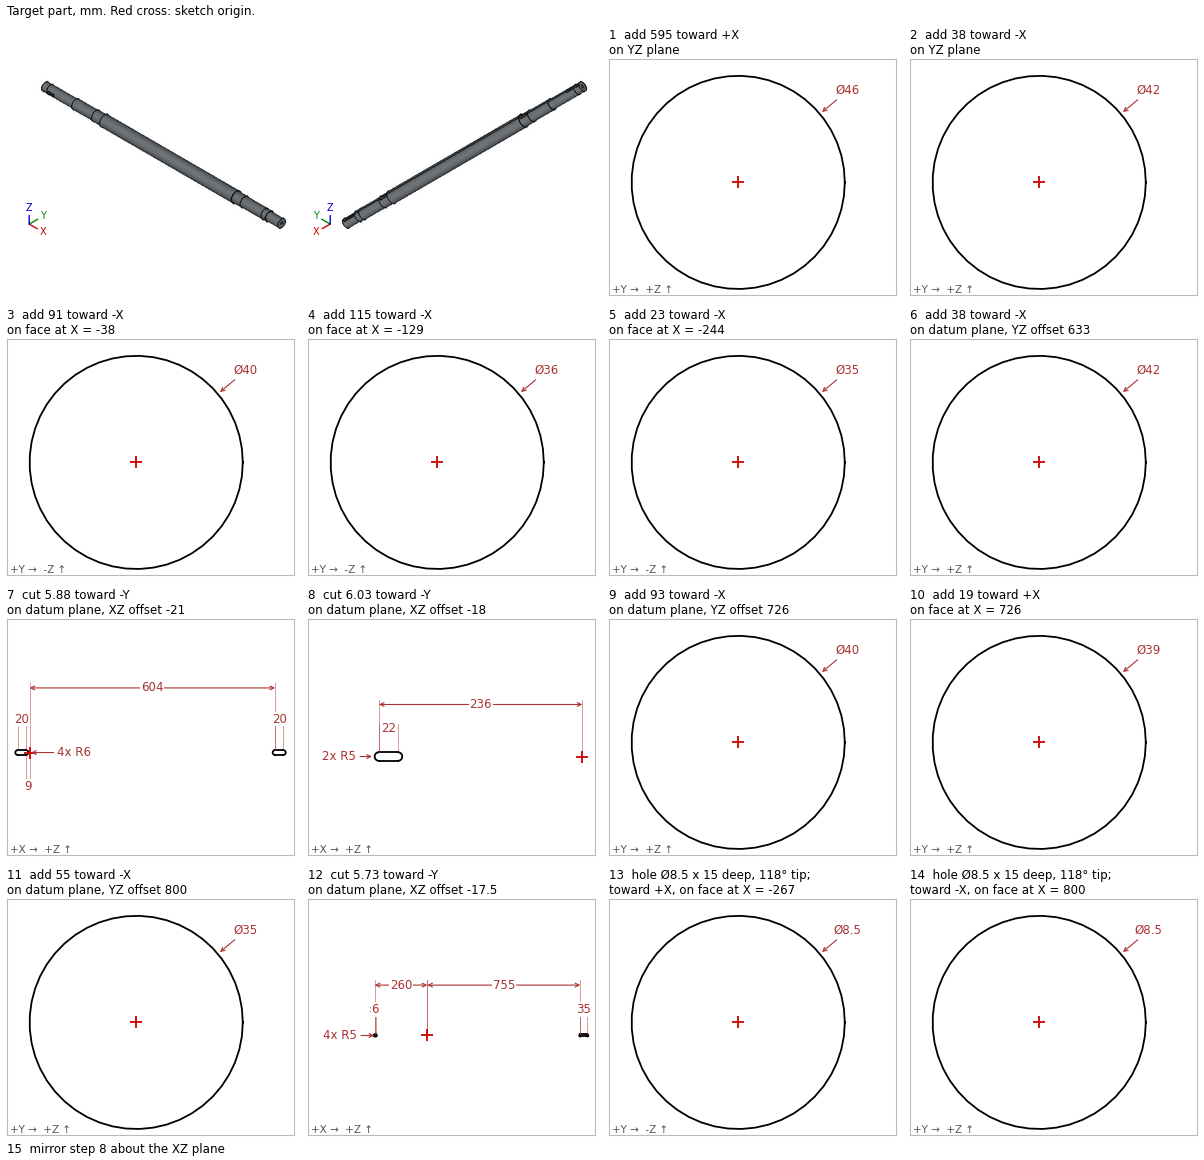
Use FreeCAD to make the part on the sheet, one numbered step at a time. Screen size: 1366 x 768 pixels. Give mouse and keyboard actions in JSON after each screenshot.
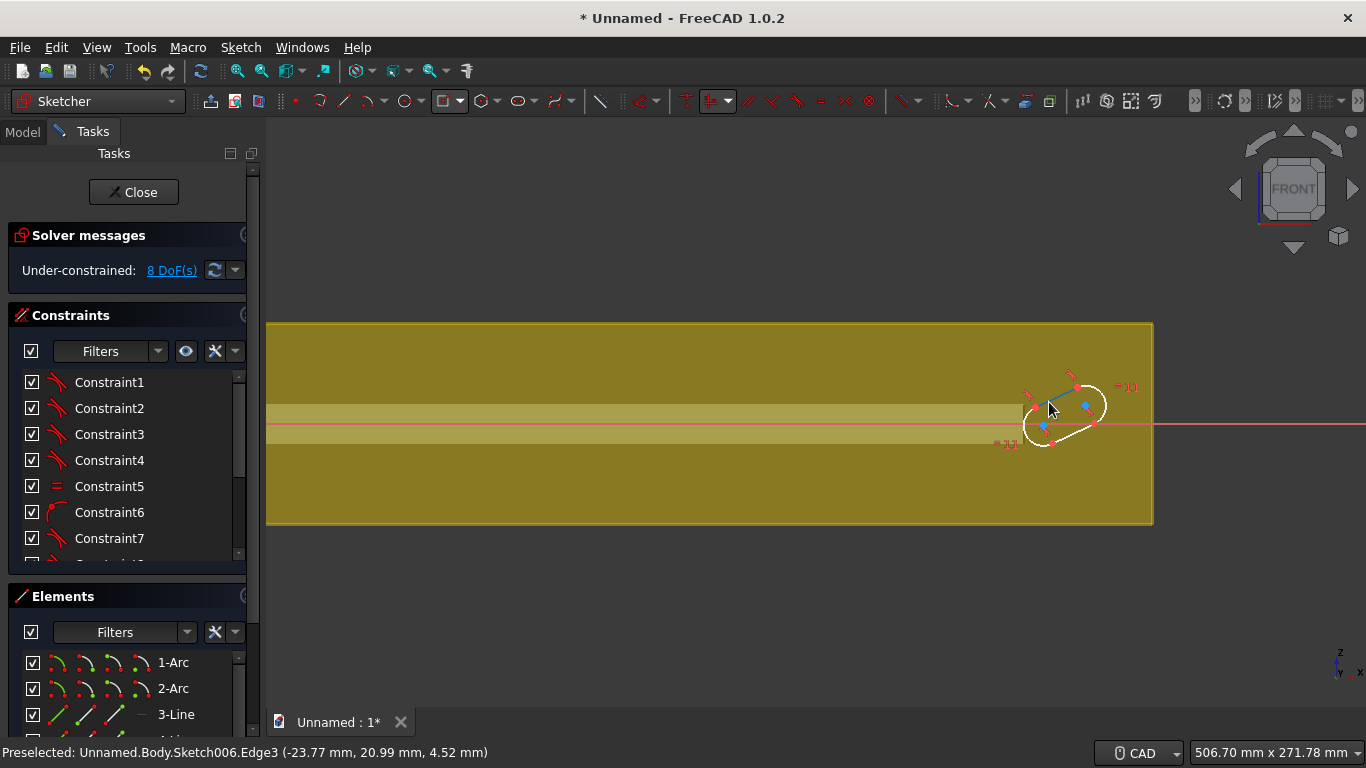
{"action": "left_click", "coordinate": [1048, 402]}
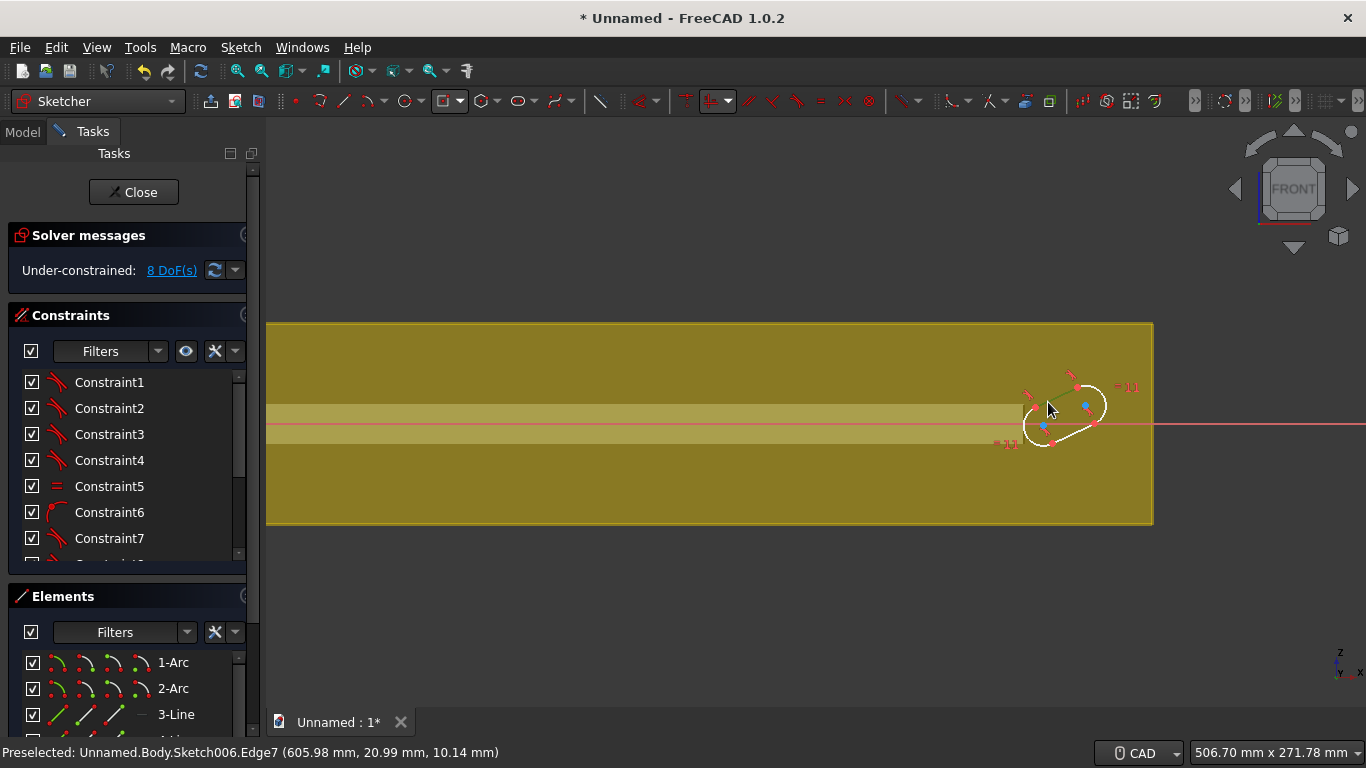
{"action": "key", "text": "h"}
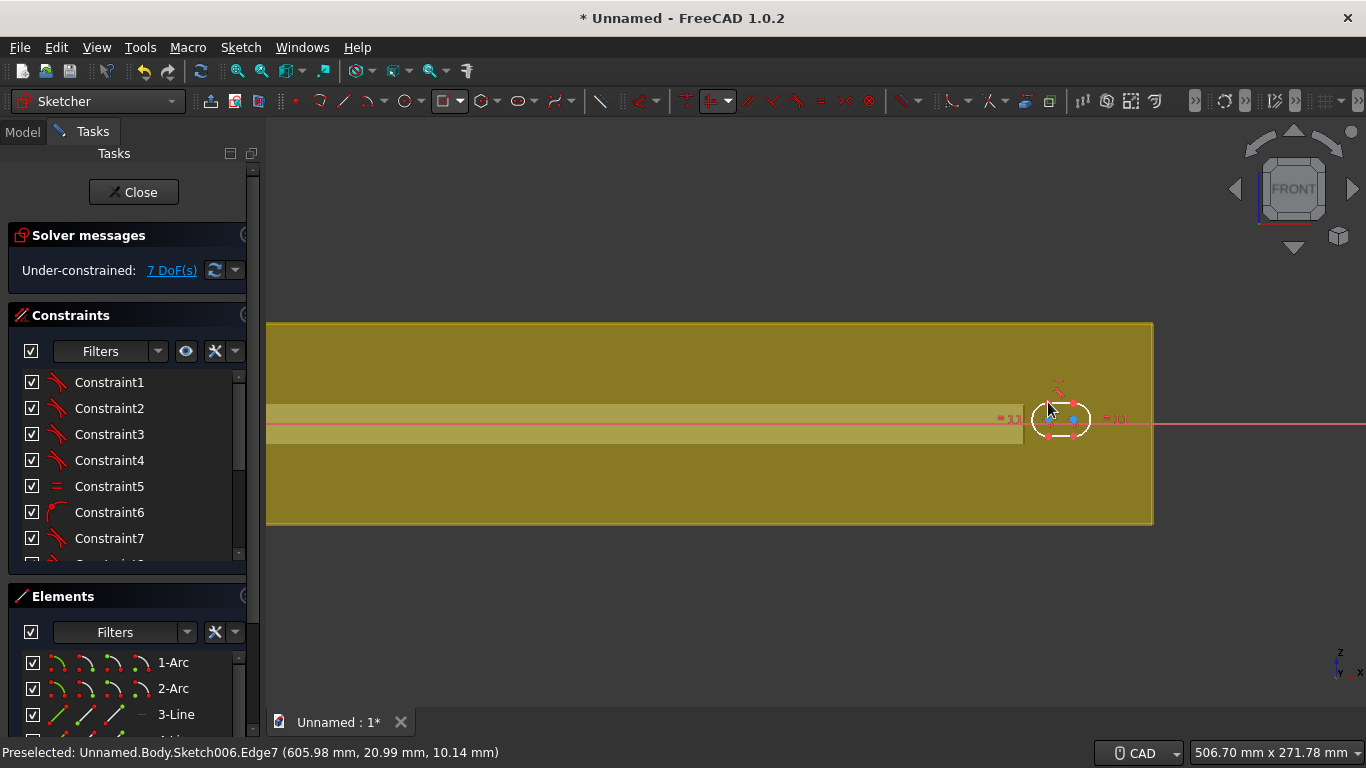
{"action": "scroll", "coordinate": [1049, 402], "scroll_direction": "down", "scroll_amount": 4}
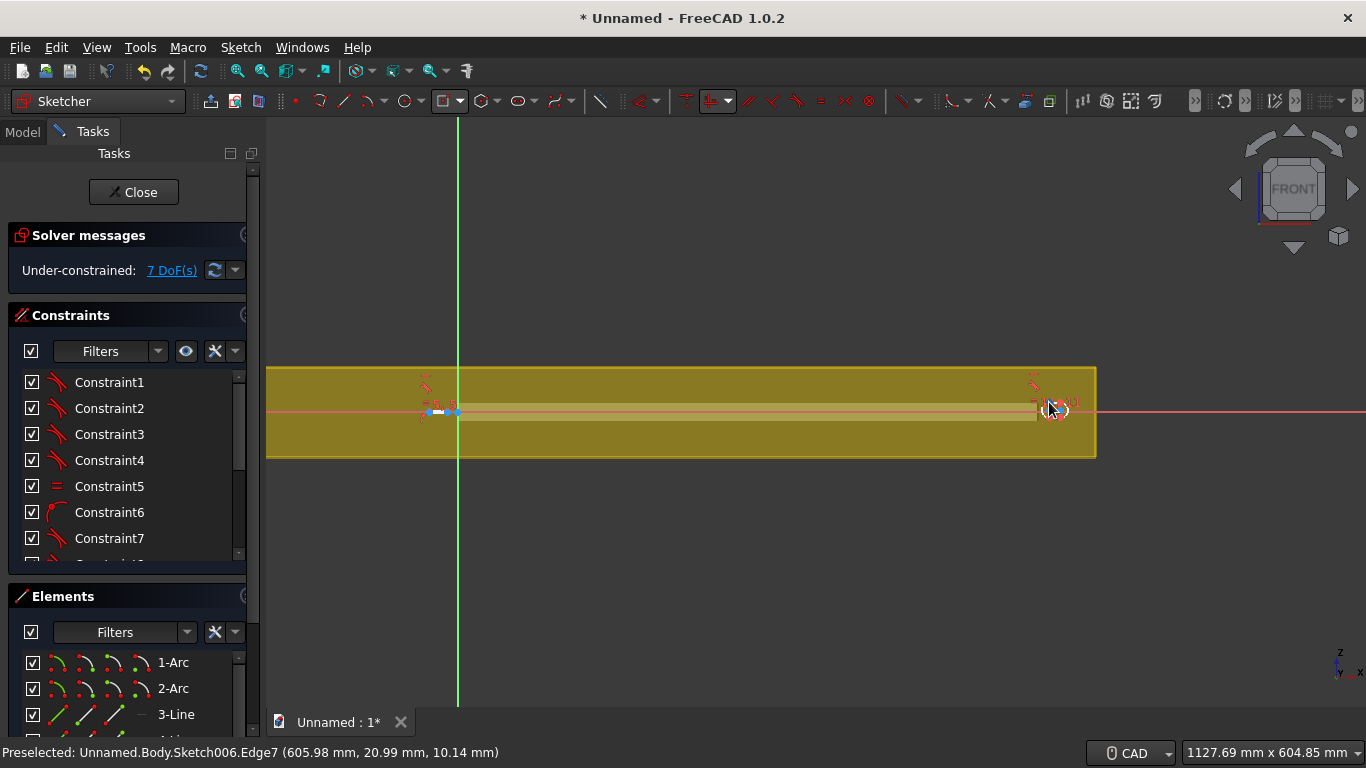
{"action": "scroll", "coordinate": [429, 412], "scroll_direction": "up", "scroll_amount": 14}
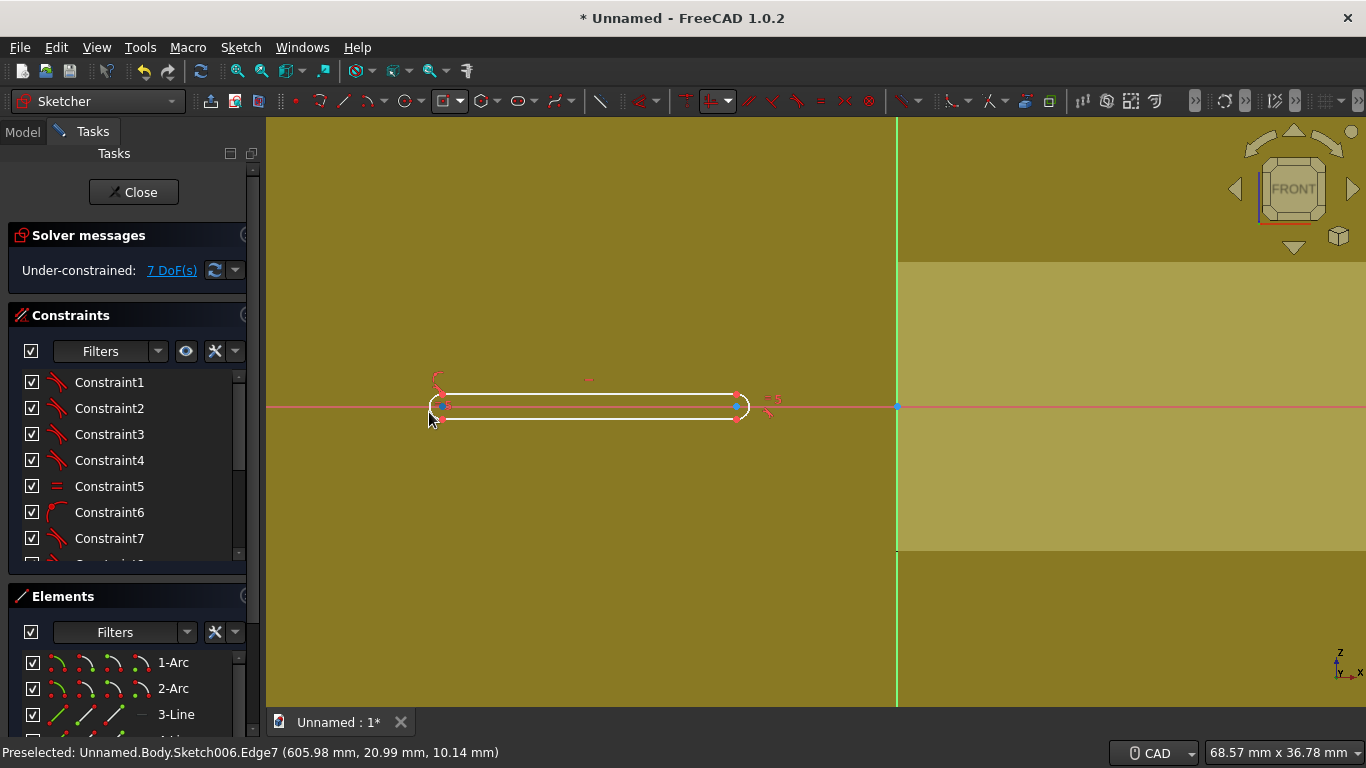
{"action": "left_click", "coordinate": [430, 407]}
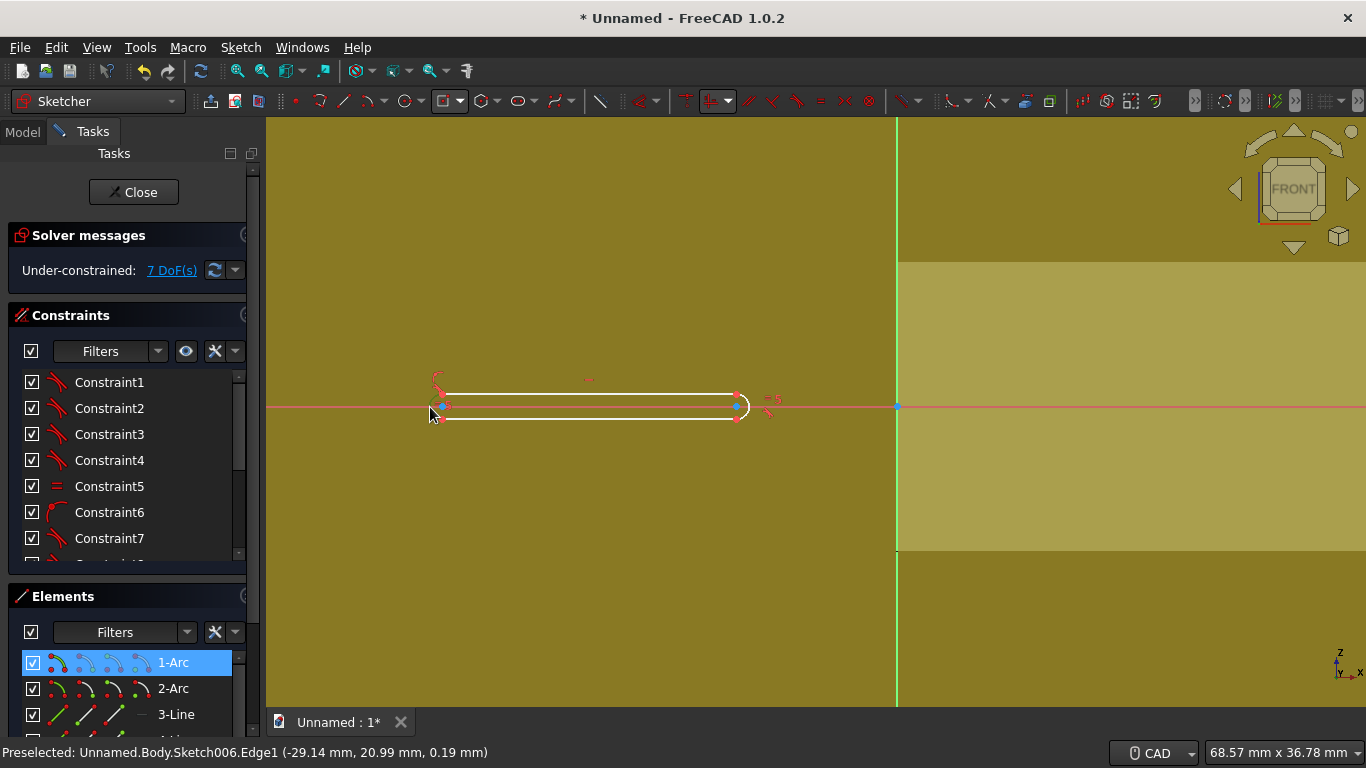
{"action": "scroll", "coordinate": [429, 412], "scroll_direction": "down", "scroll_amount": 14}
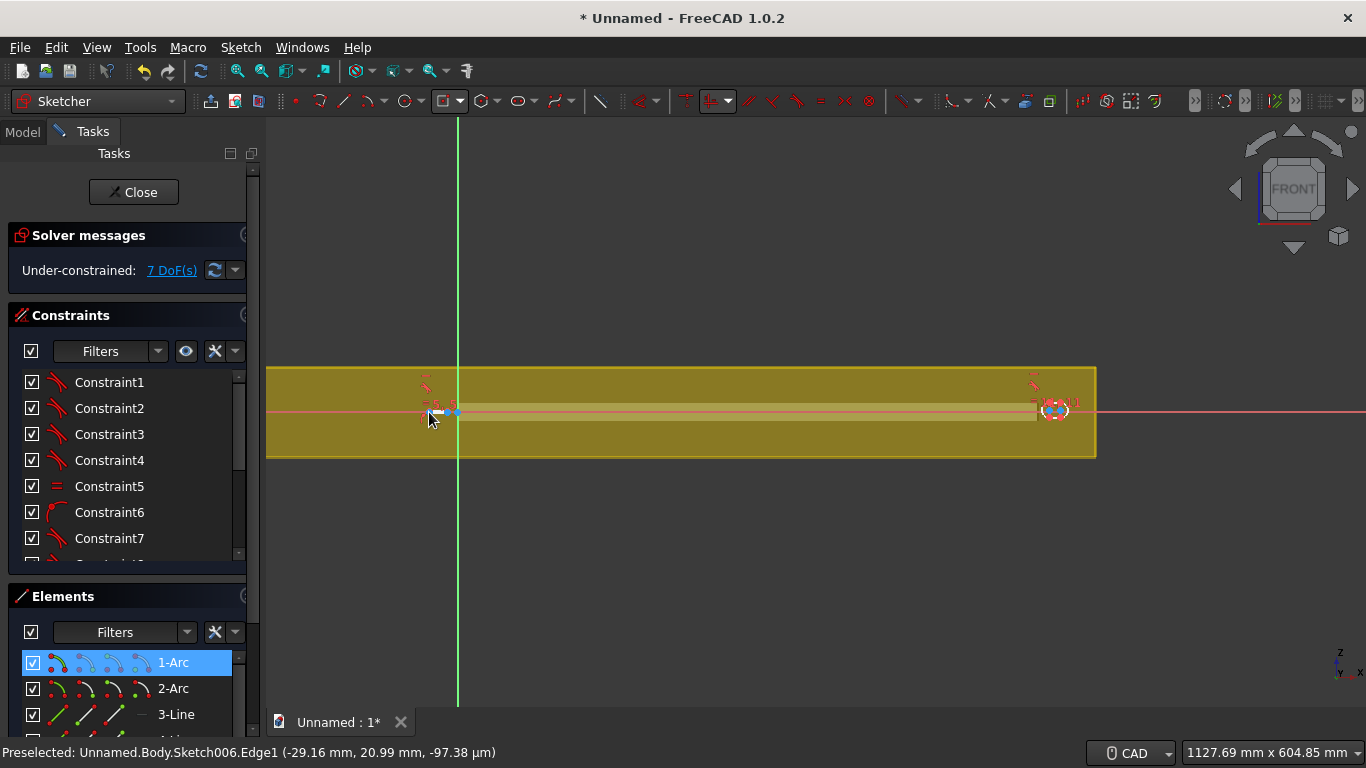
{"action": "scroll", "coordinate": [1043, 406], "scroll_direction": "up", "scroll_amount": 4}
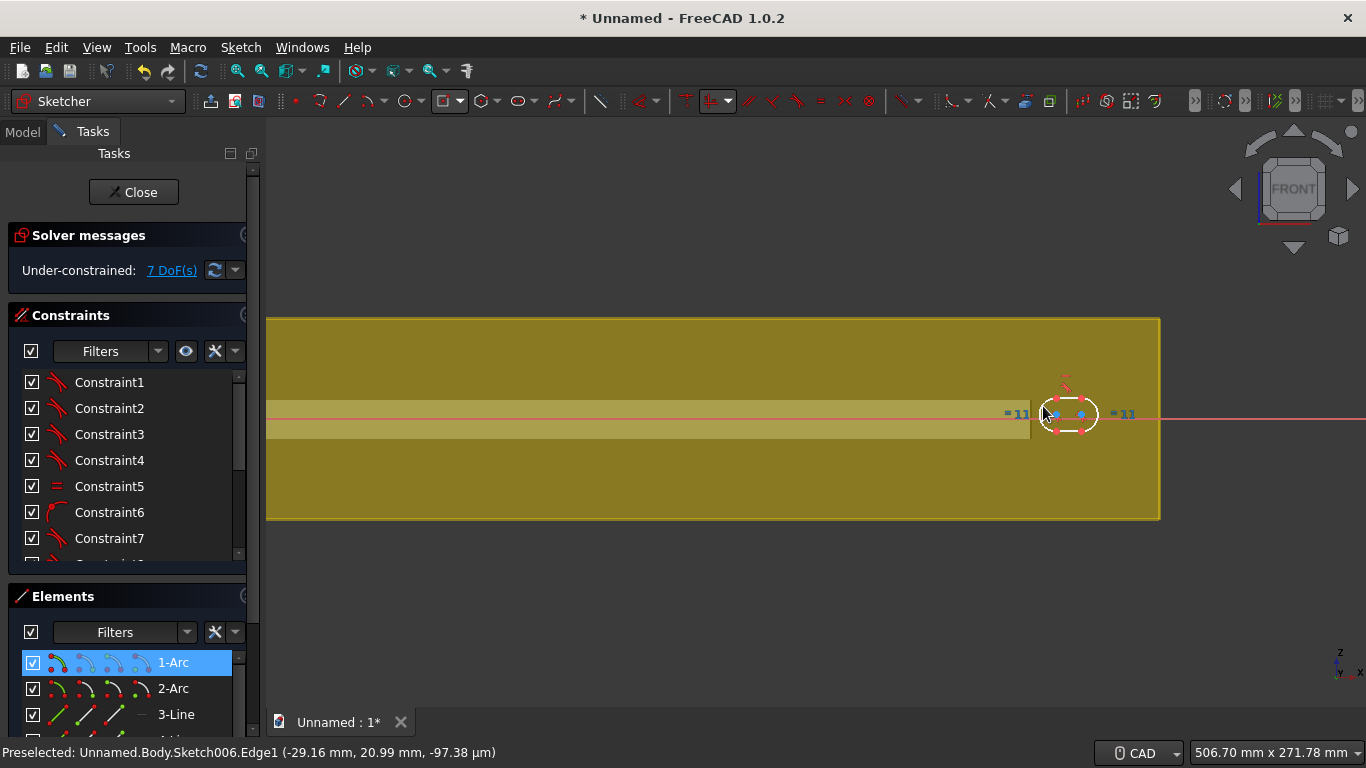
{"action": "left_click", "coordinate": [1043, 405]}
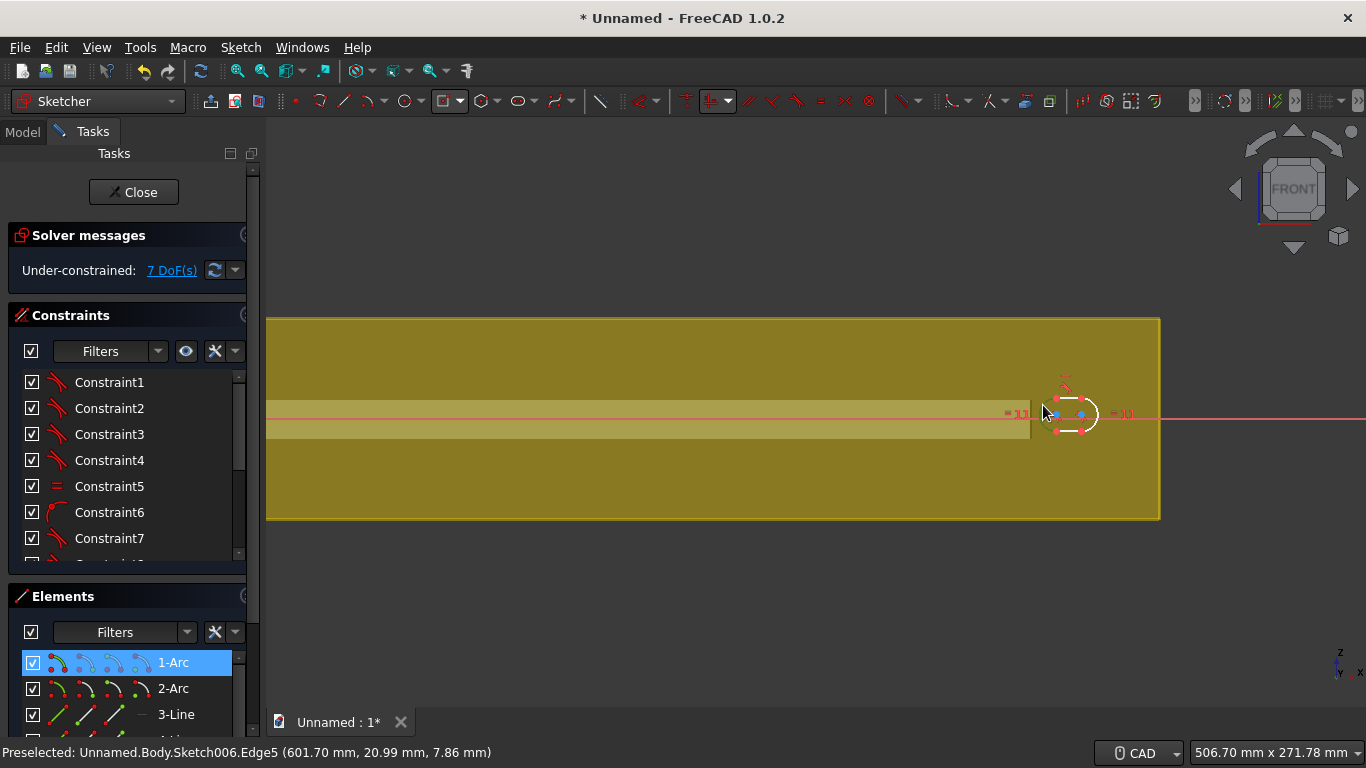
{"action": "left_click", "coordinate": [822, 102]}